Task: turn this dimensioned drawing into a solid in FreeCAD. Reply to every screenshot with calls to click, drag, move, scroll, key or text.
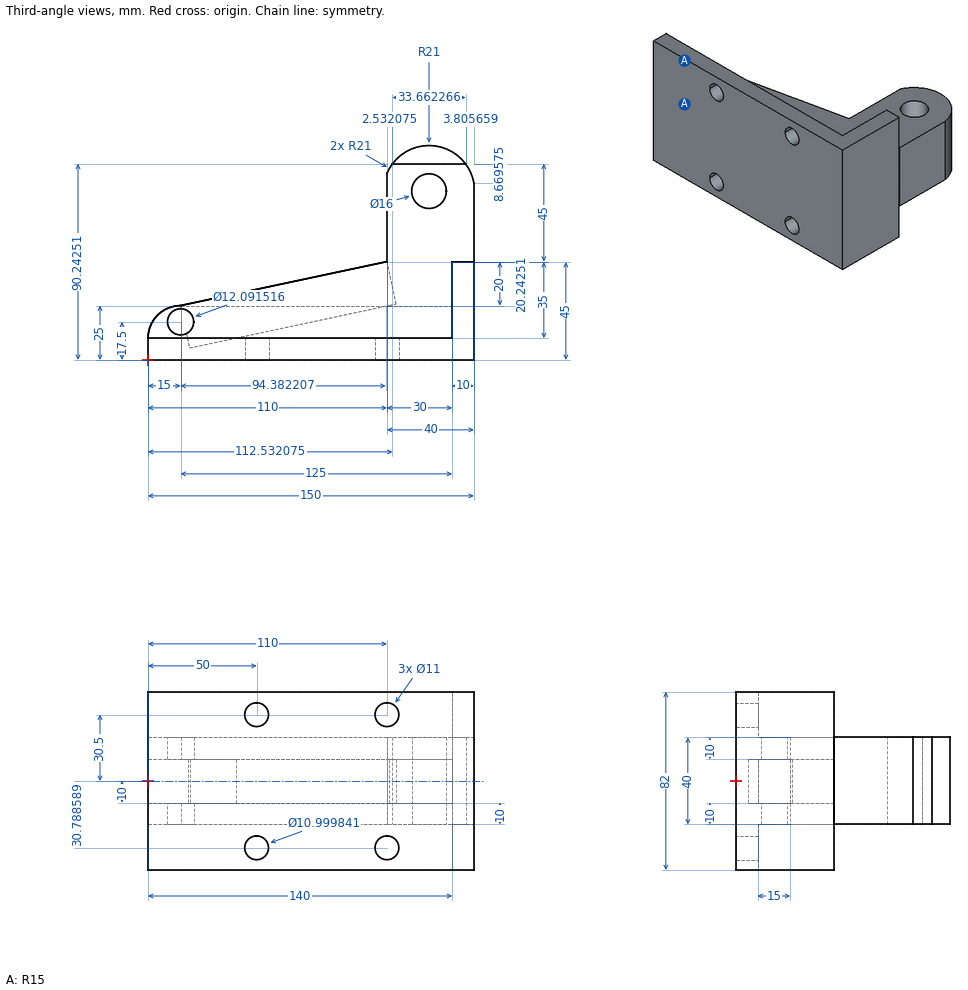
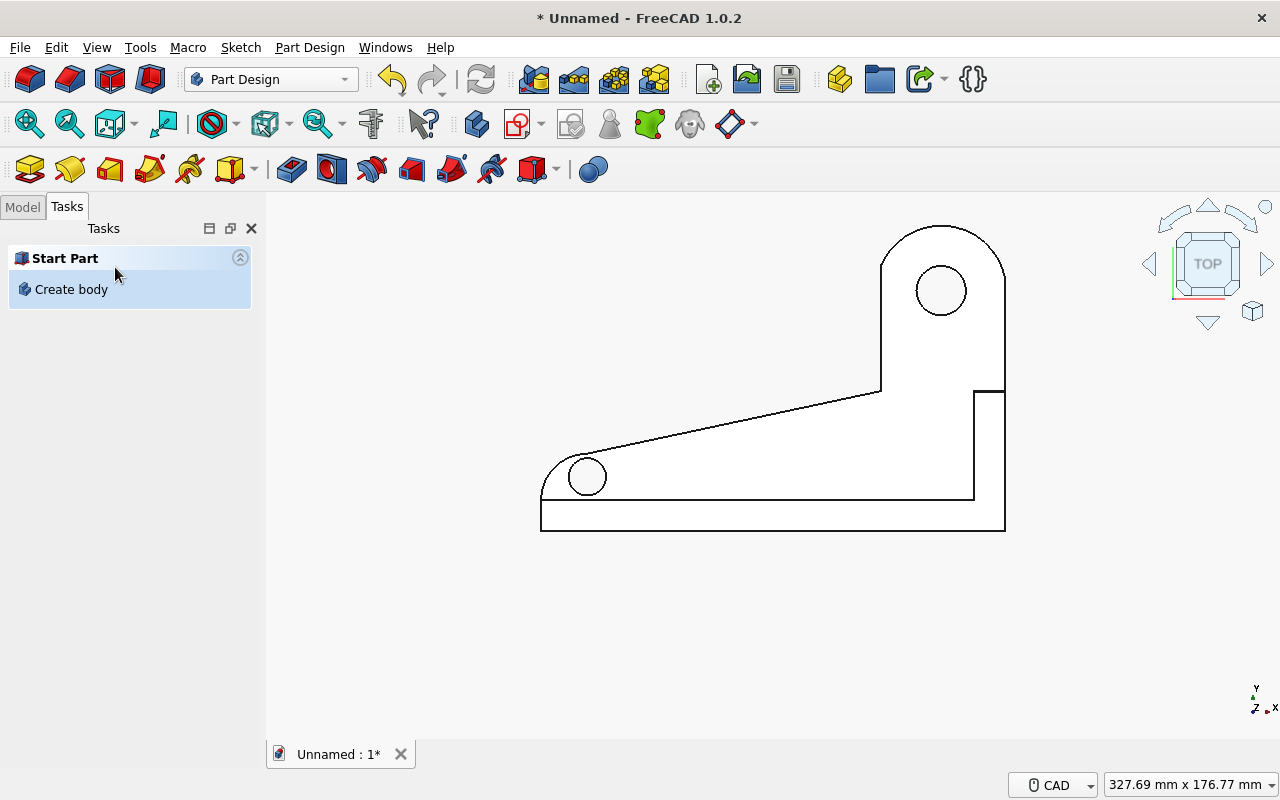
key(4)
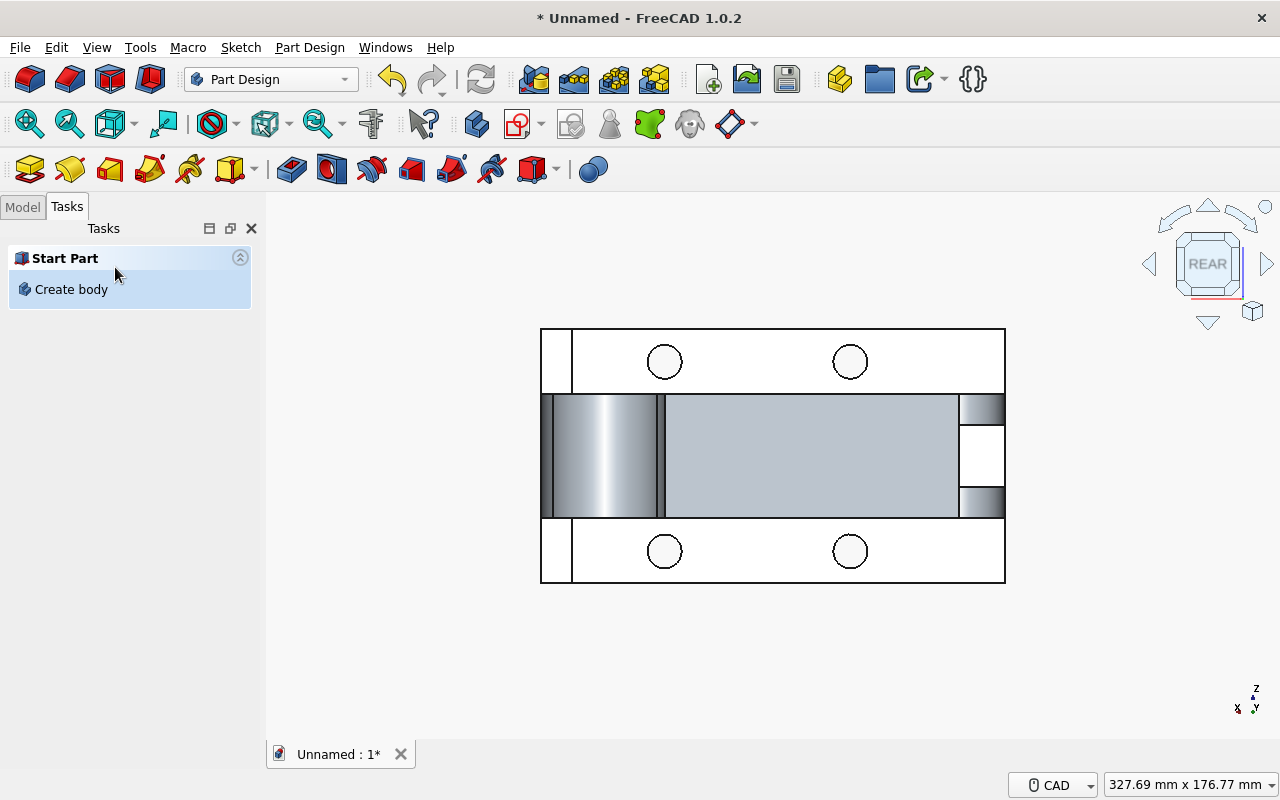
click(728, 455)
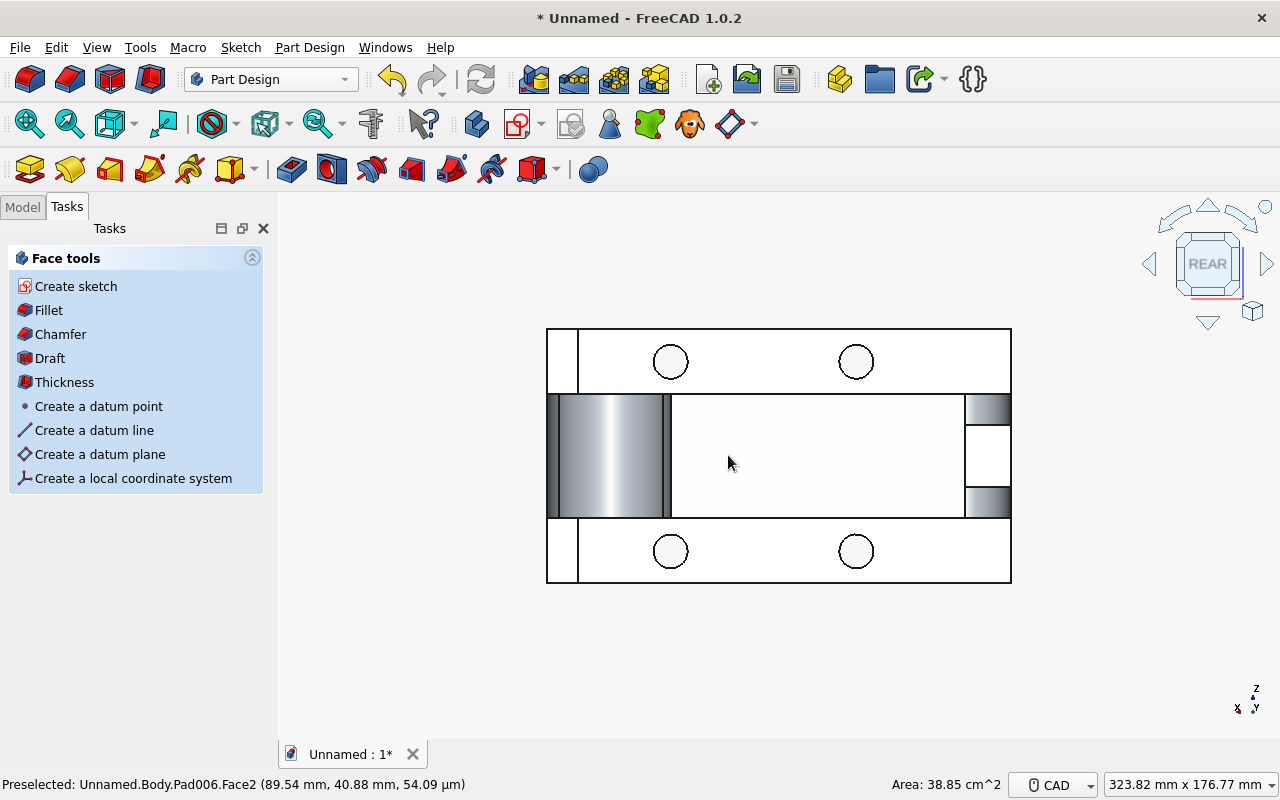
click(518, 124)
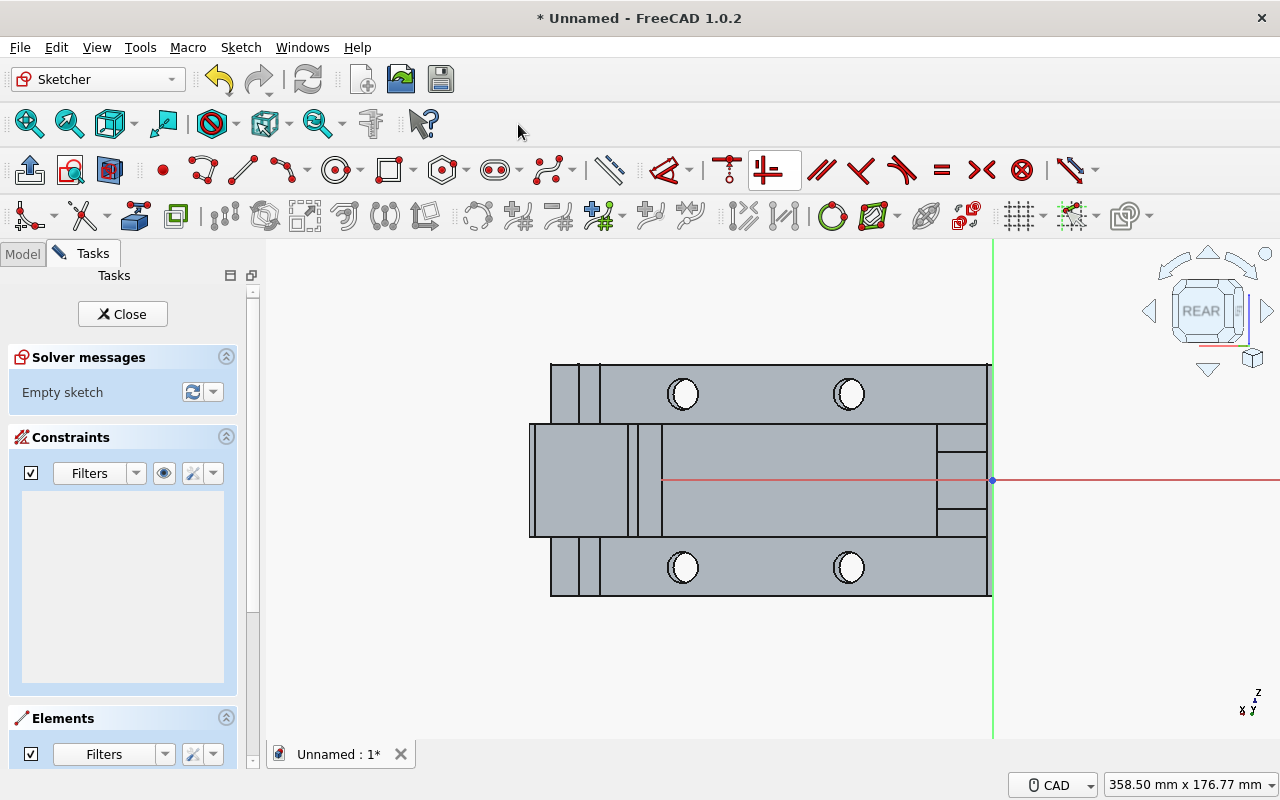
scroll(977, 470, up, 3)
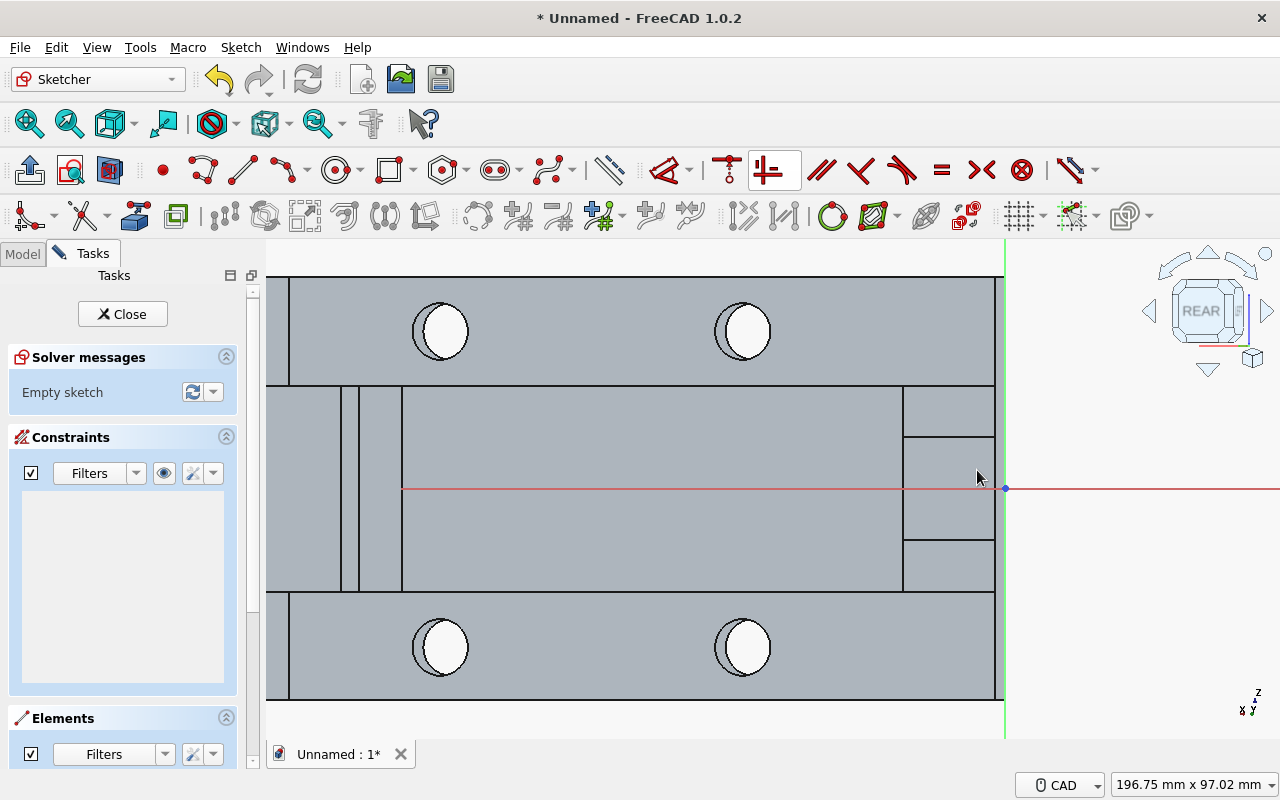
key(g)
key(r)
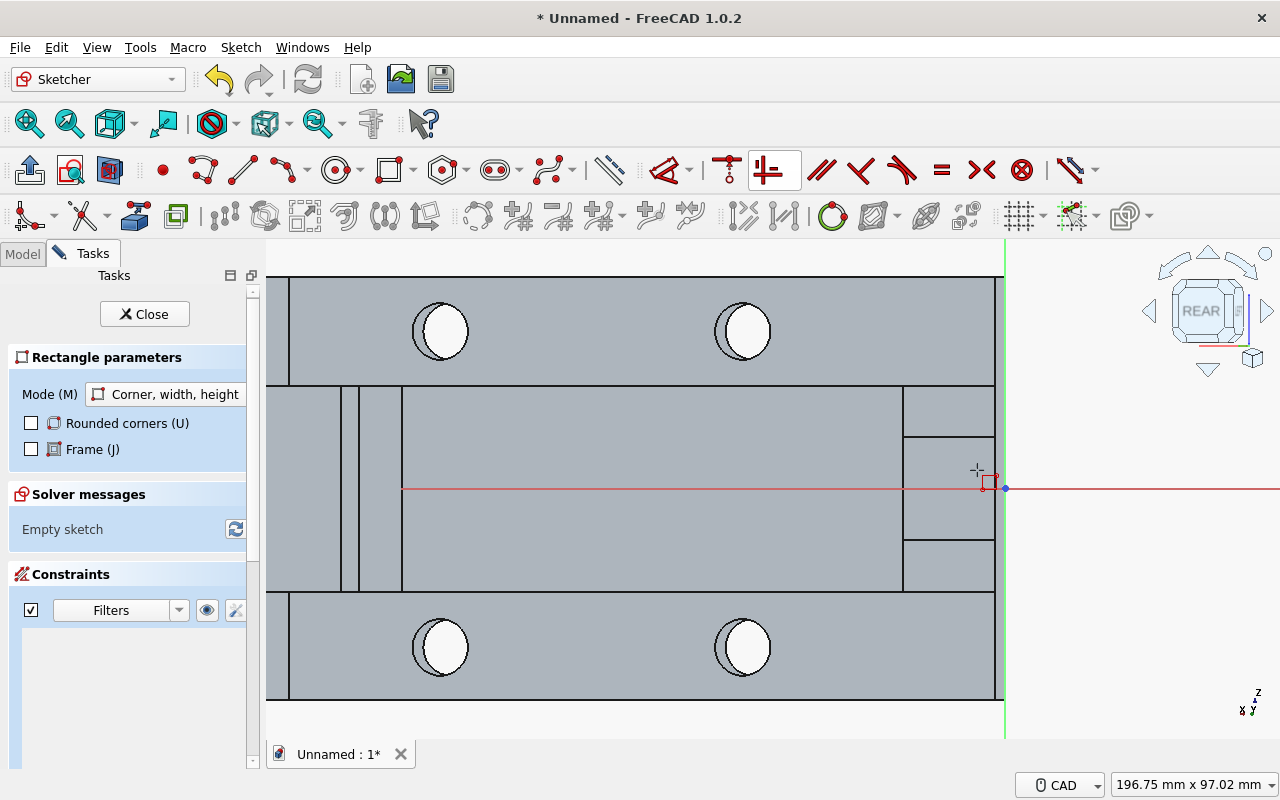
click(402, 437)
move(903, 540)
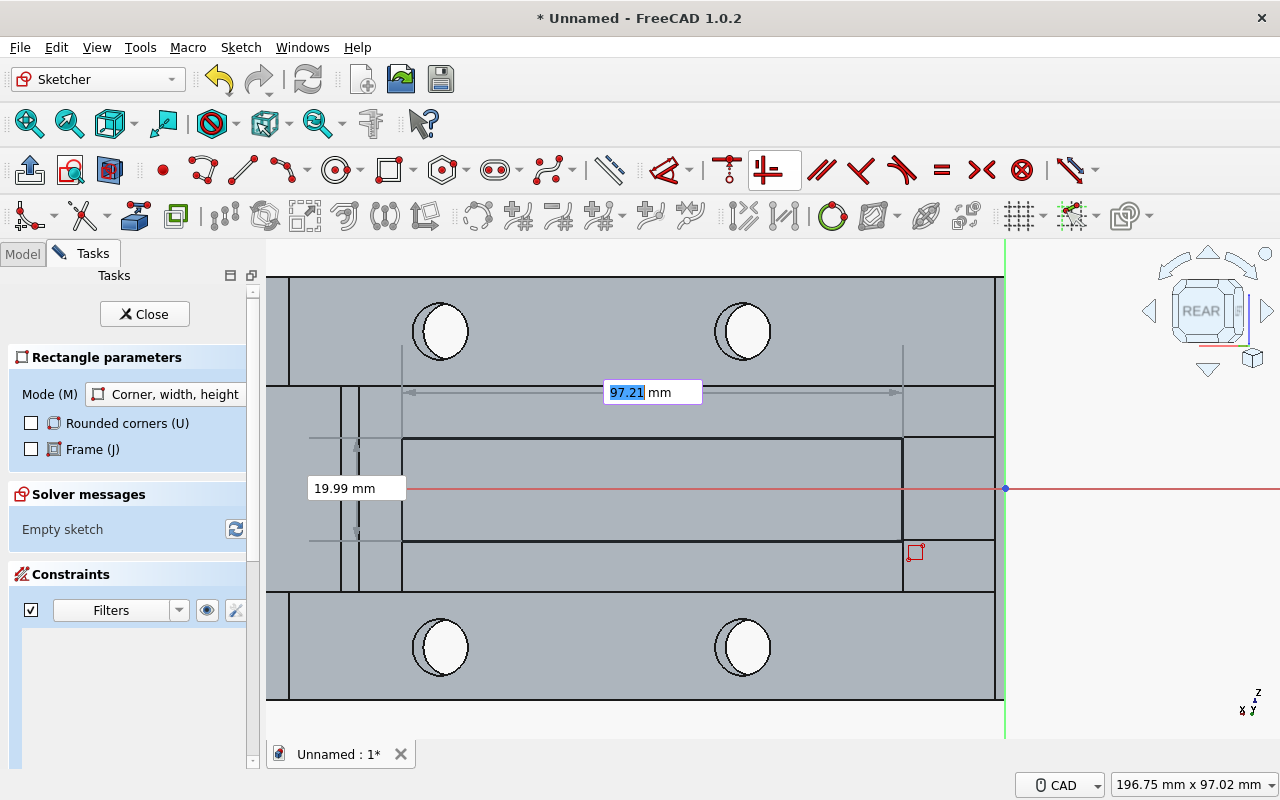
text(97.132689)
key(Tab)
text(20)
key(Return)
key(Escape)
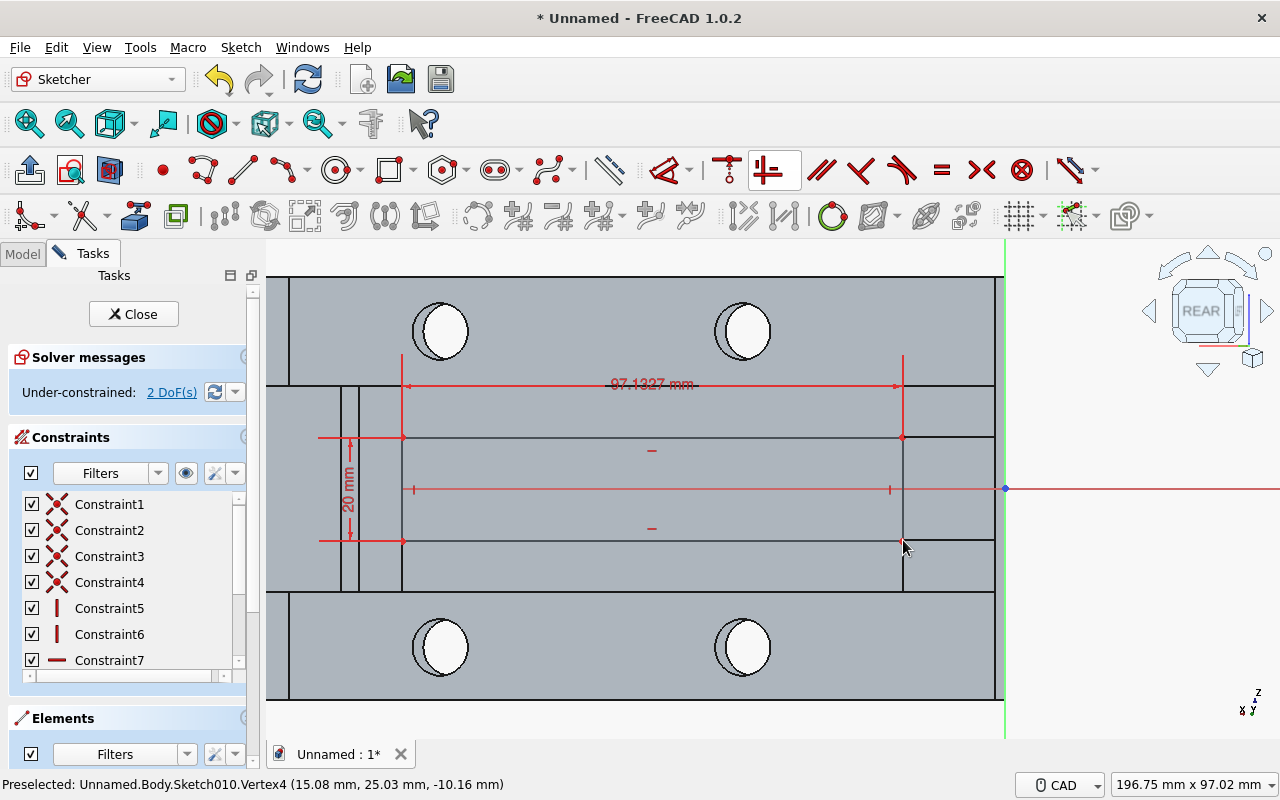
key(d)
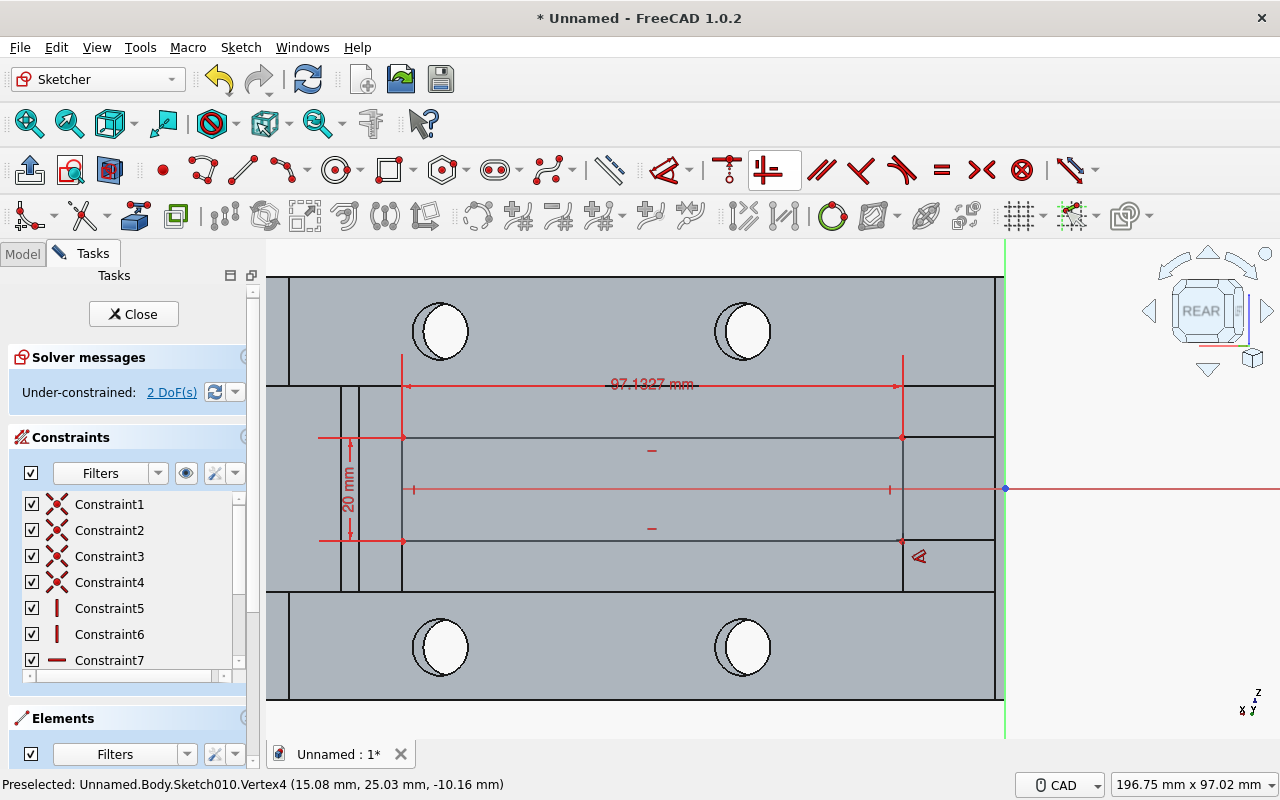
click(402, 438)
click(368, 463)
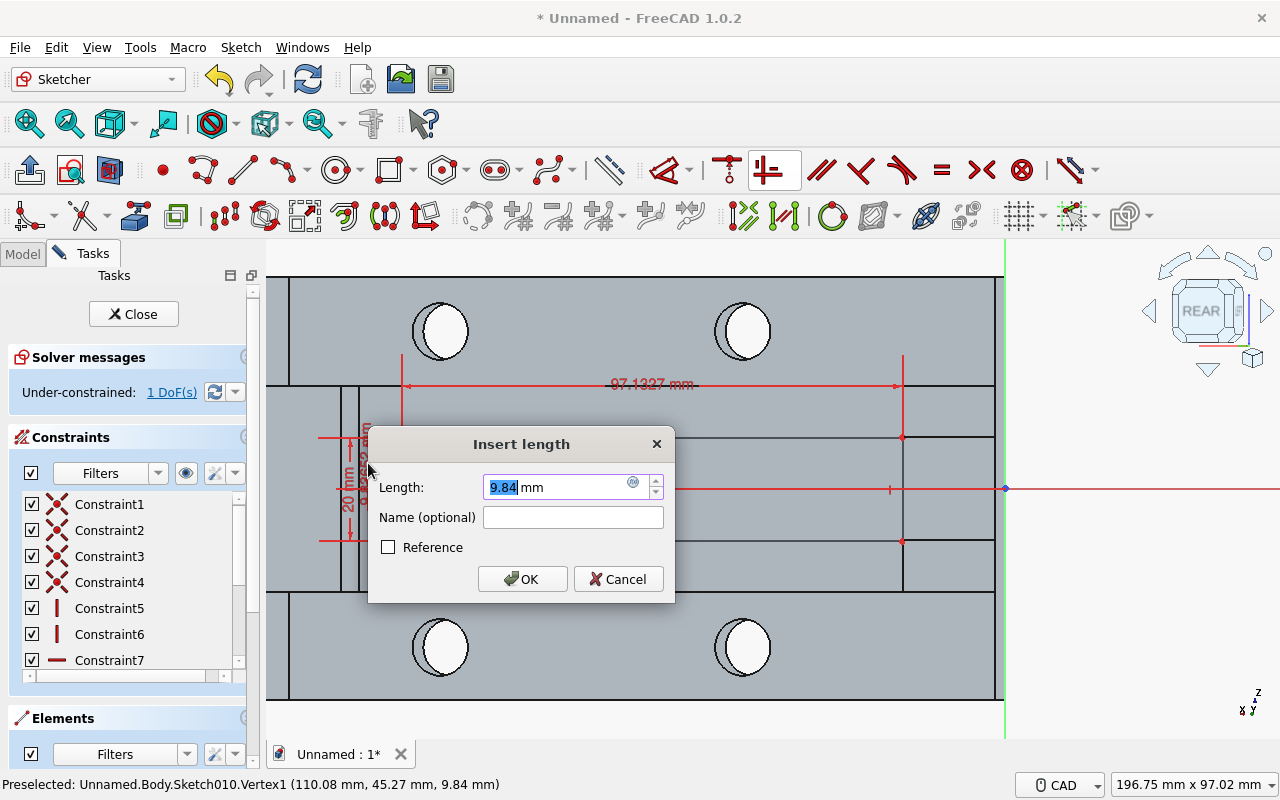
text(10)
key(Return)